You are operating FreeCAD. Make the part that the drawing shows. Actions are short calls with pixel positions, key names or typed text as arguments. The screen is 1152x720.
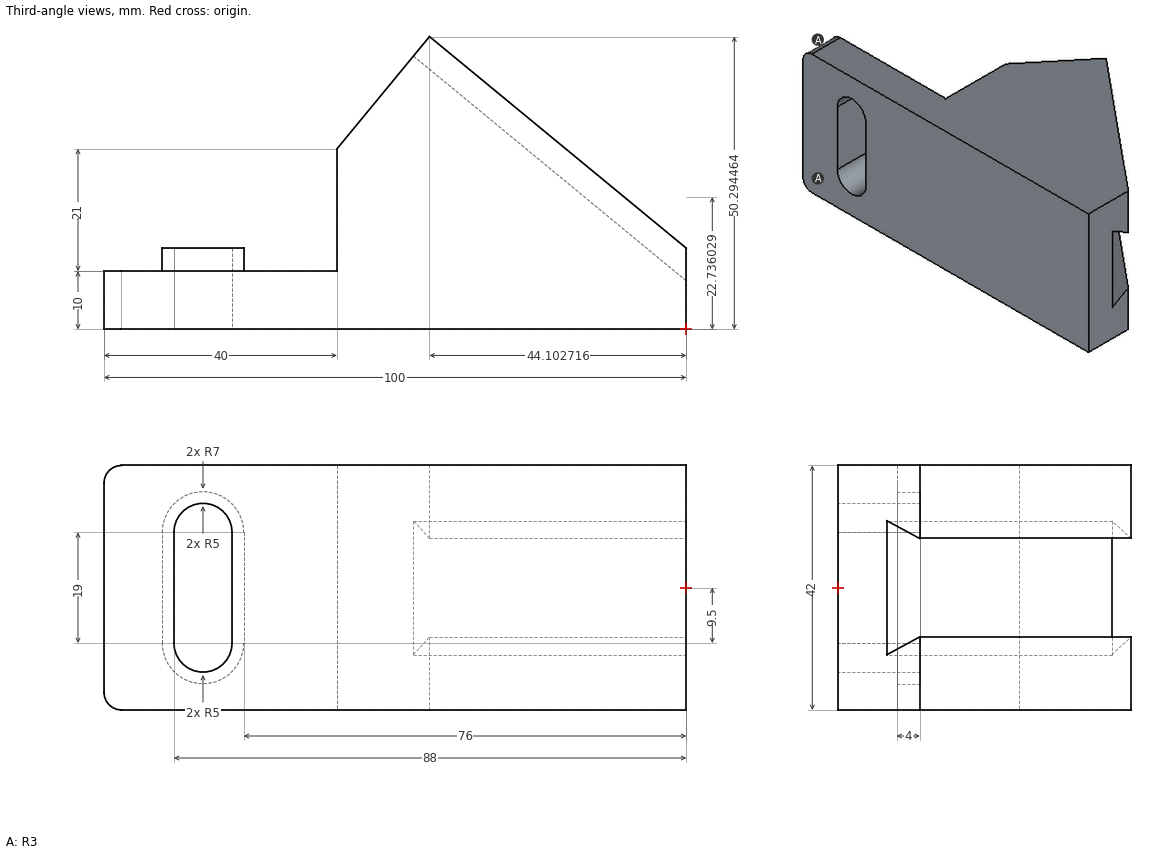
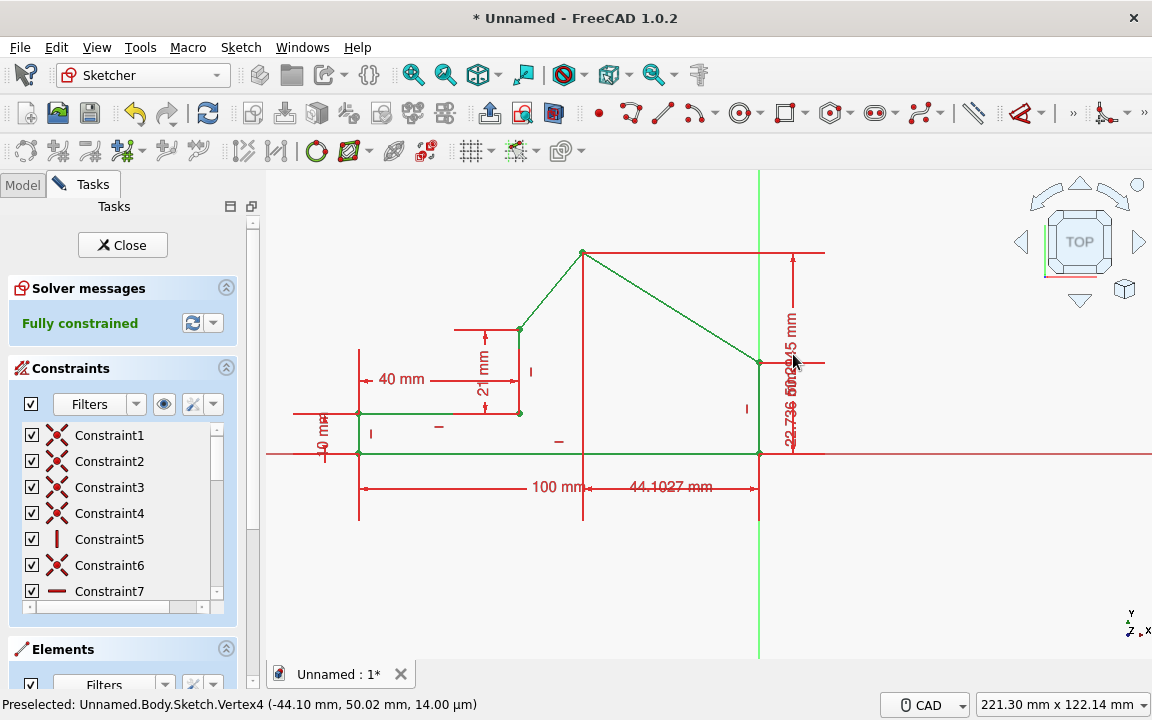
click(123, 245)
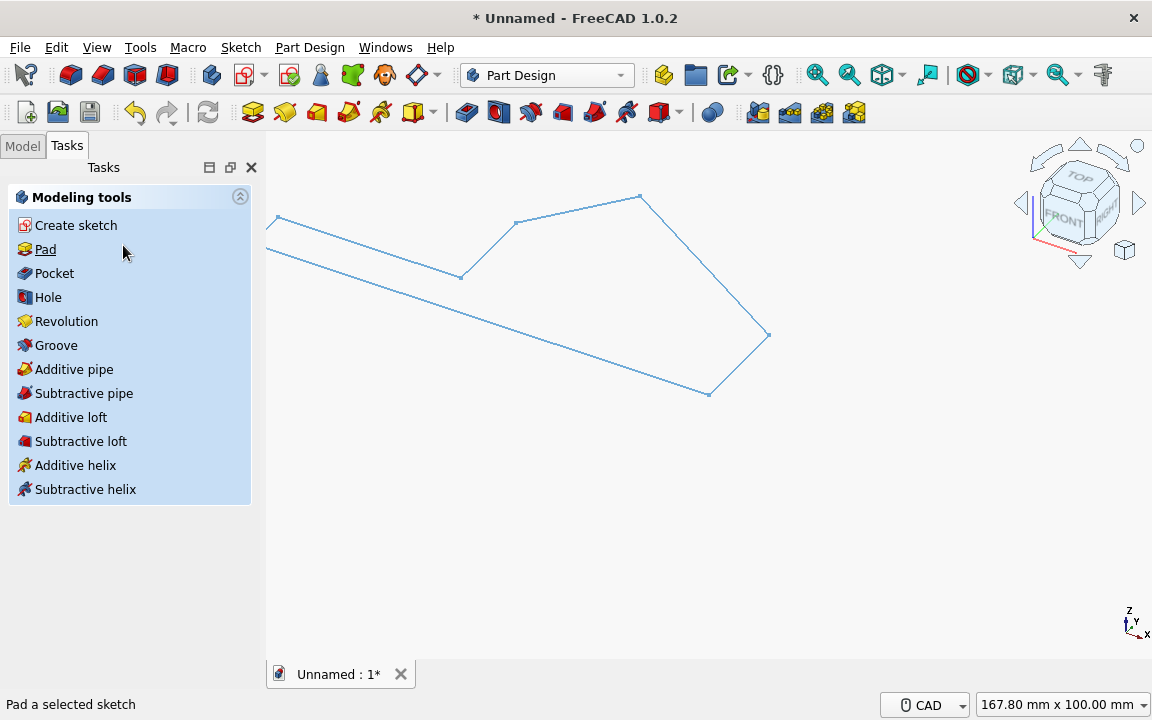
click(254, 112)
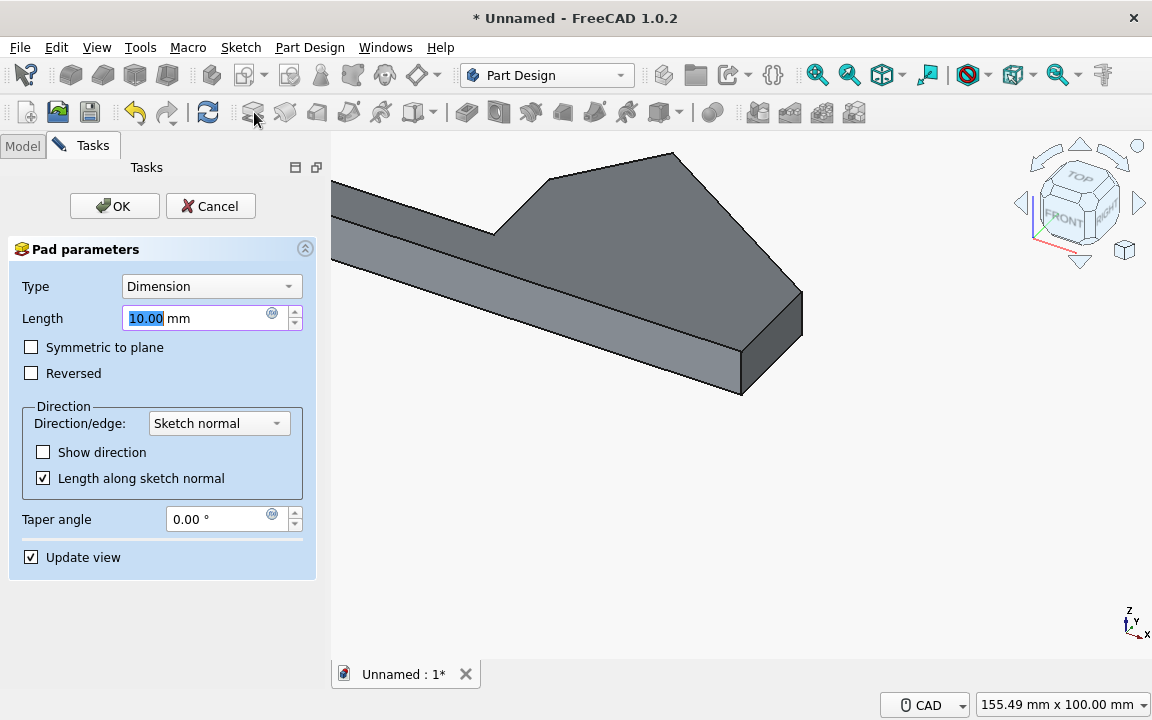
text(42)
key(Tab)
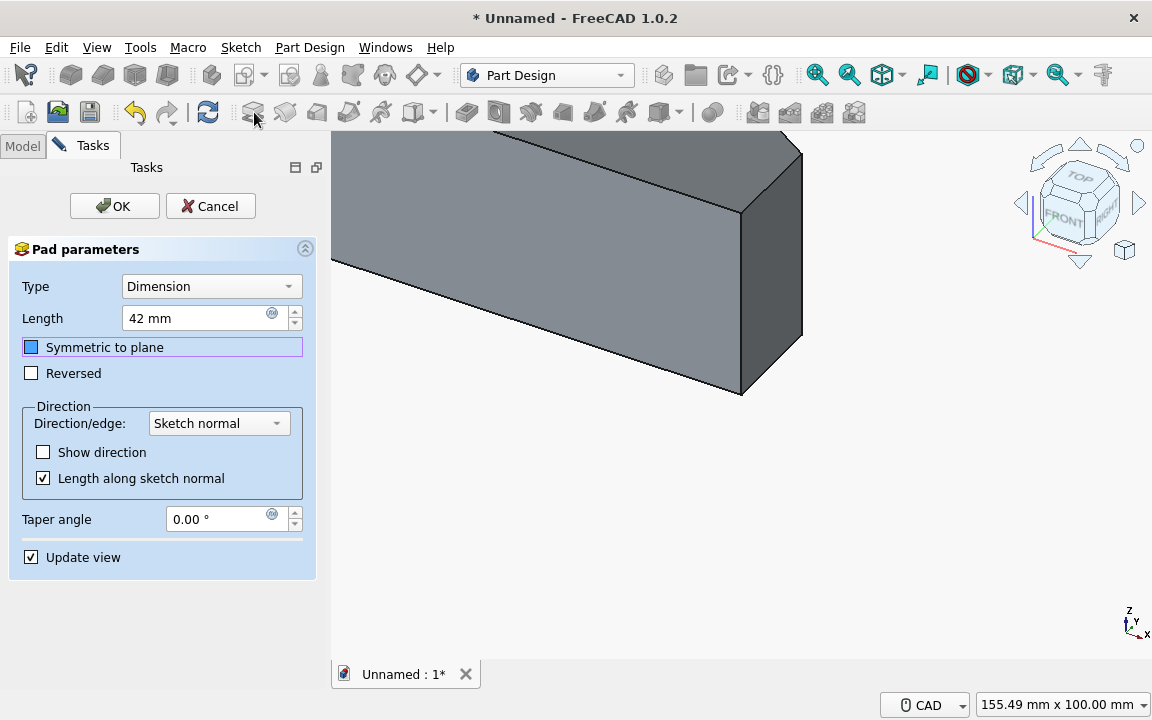
click(30, 347)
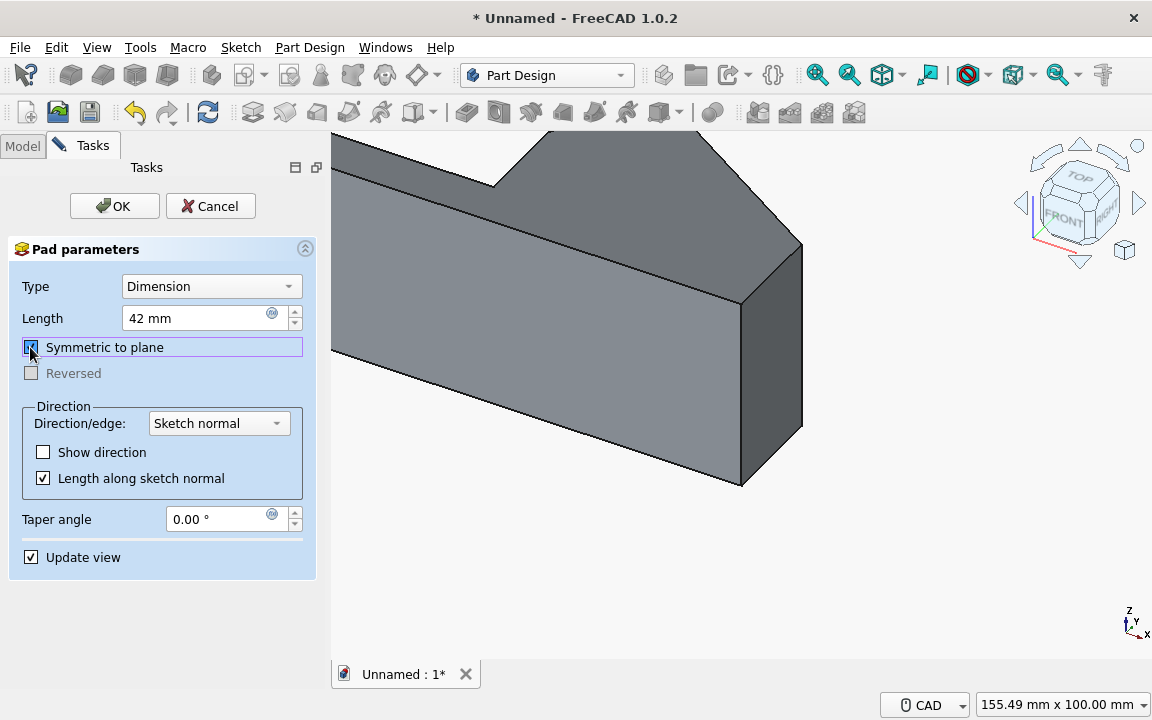
click(115, 206)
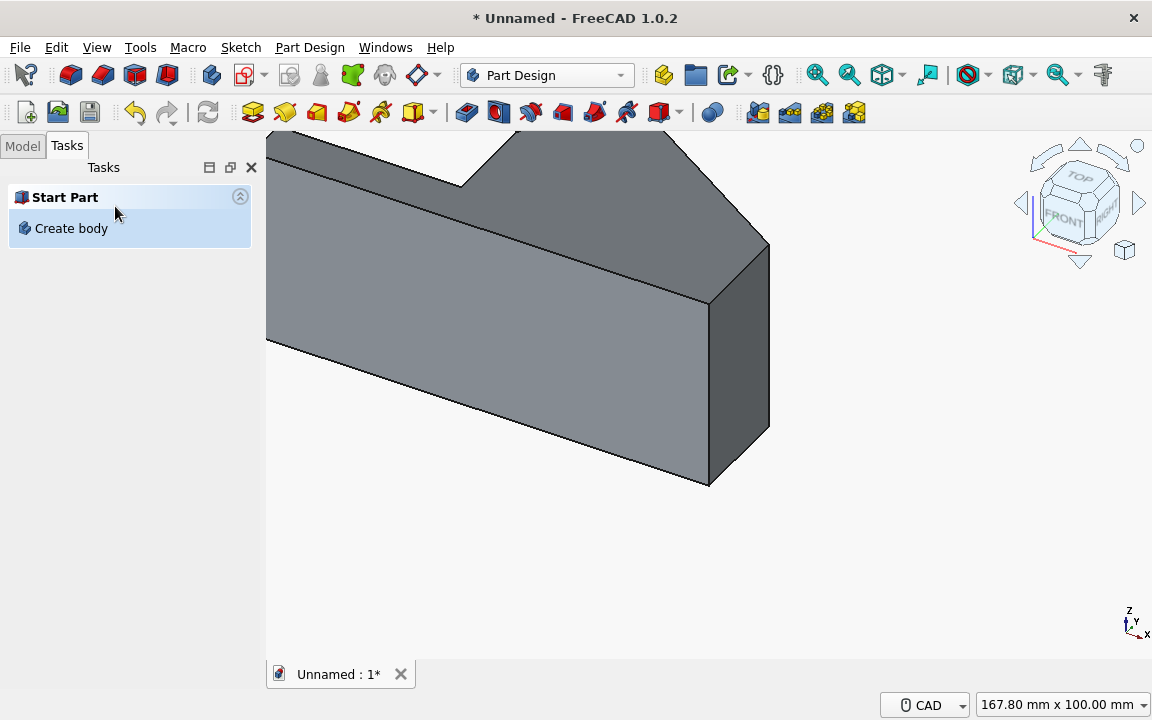
click(818, 76)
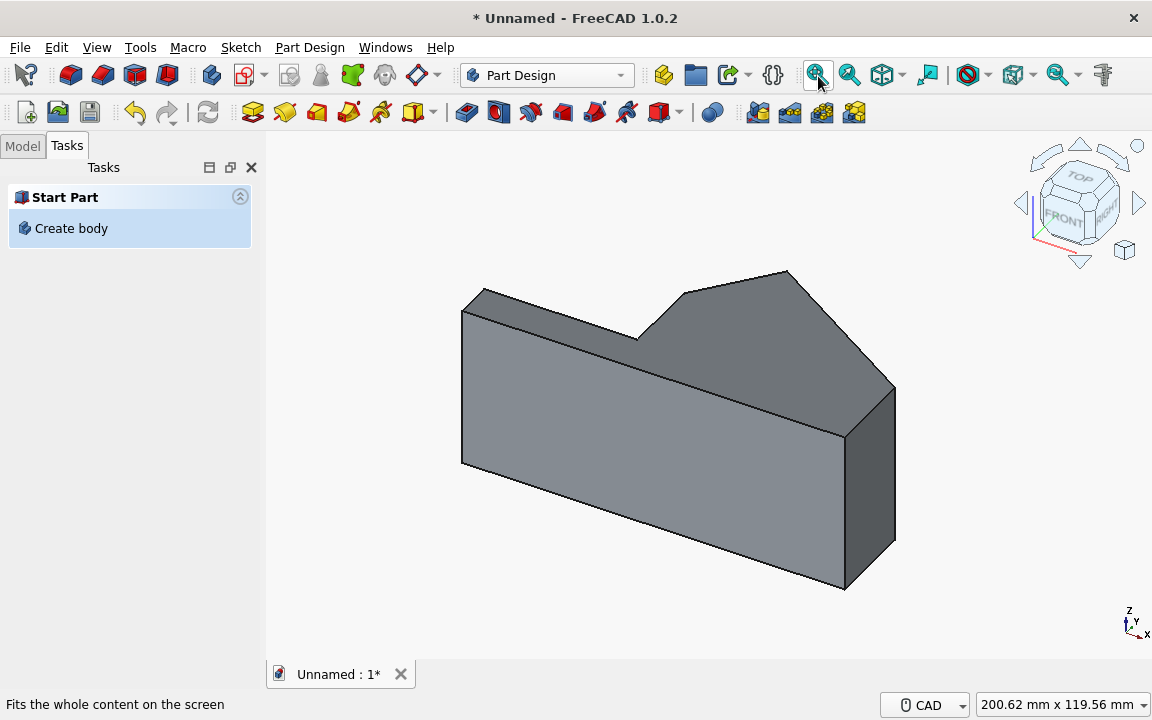
key(4)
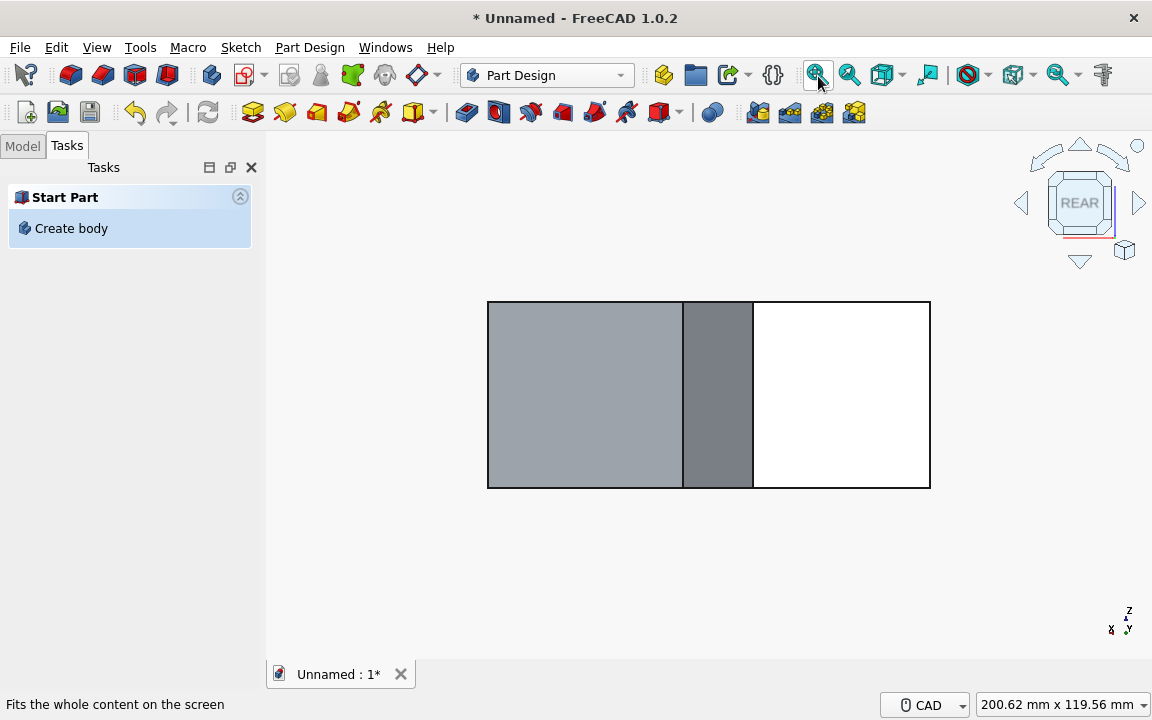
click(841, 394)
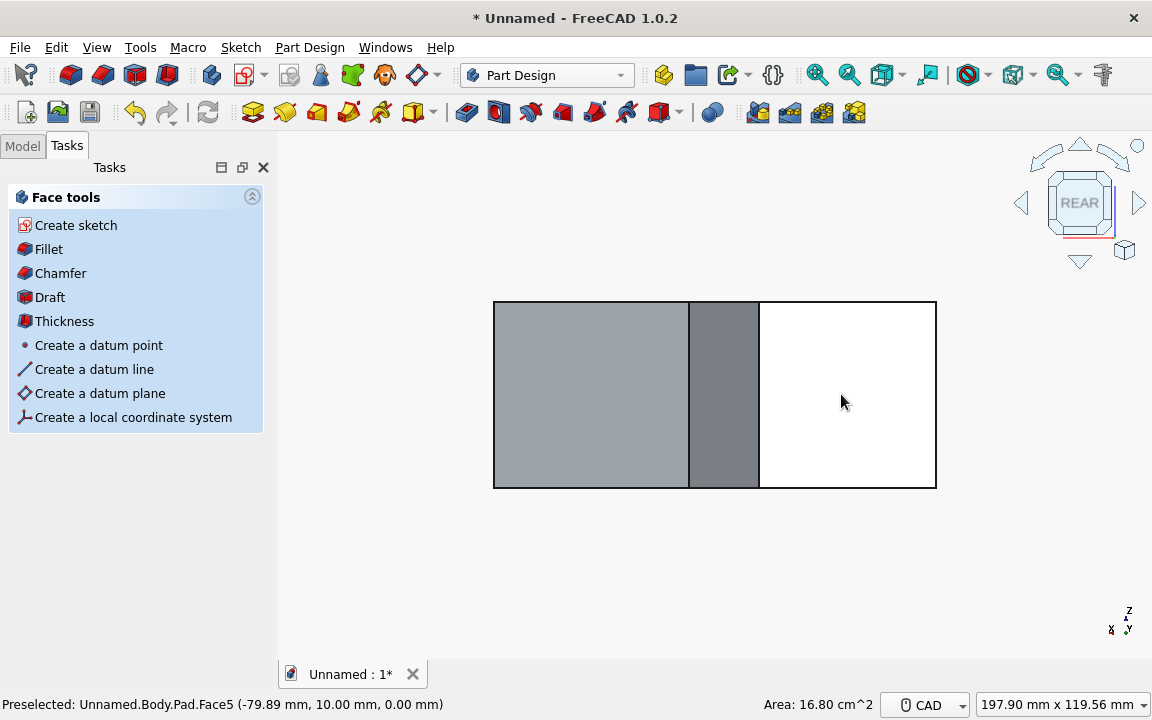
click(244, 76)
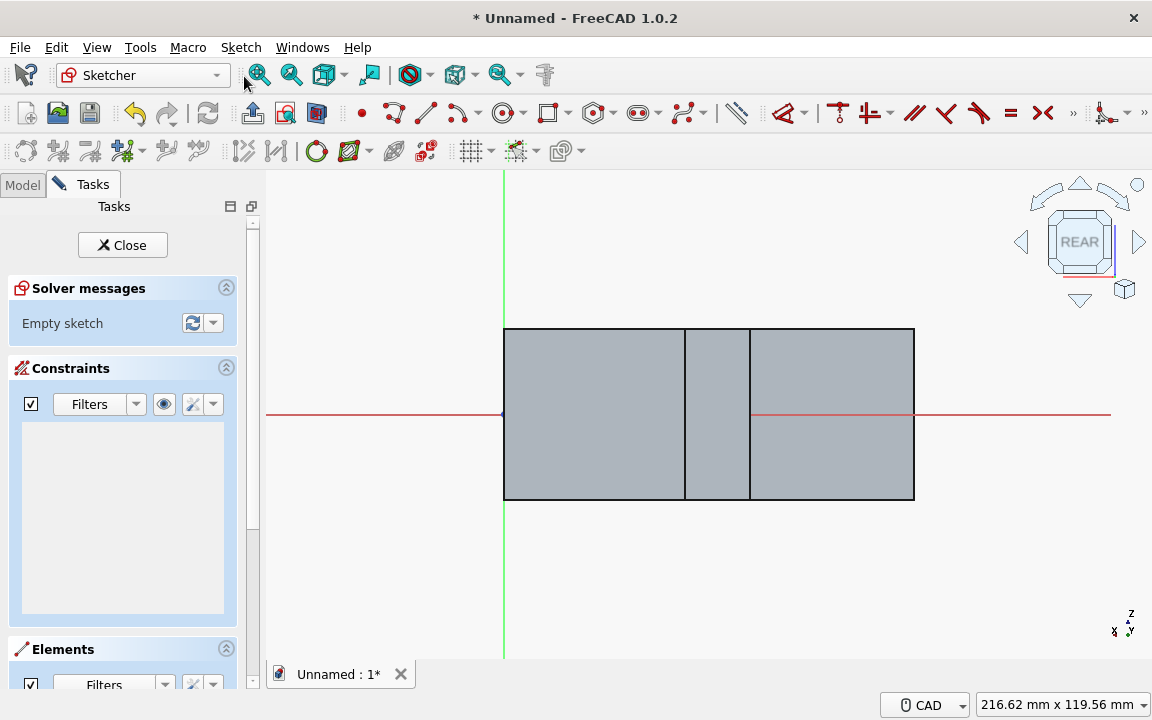
scroll(987, 414, up, 4)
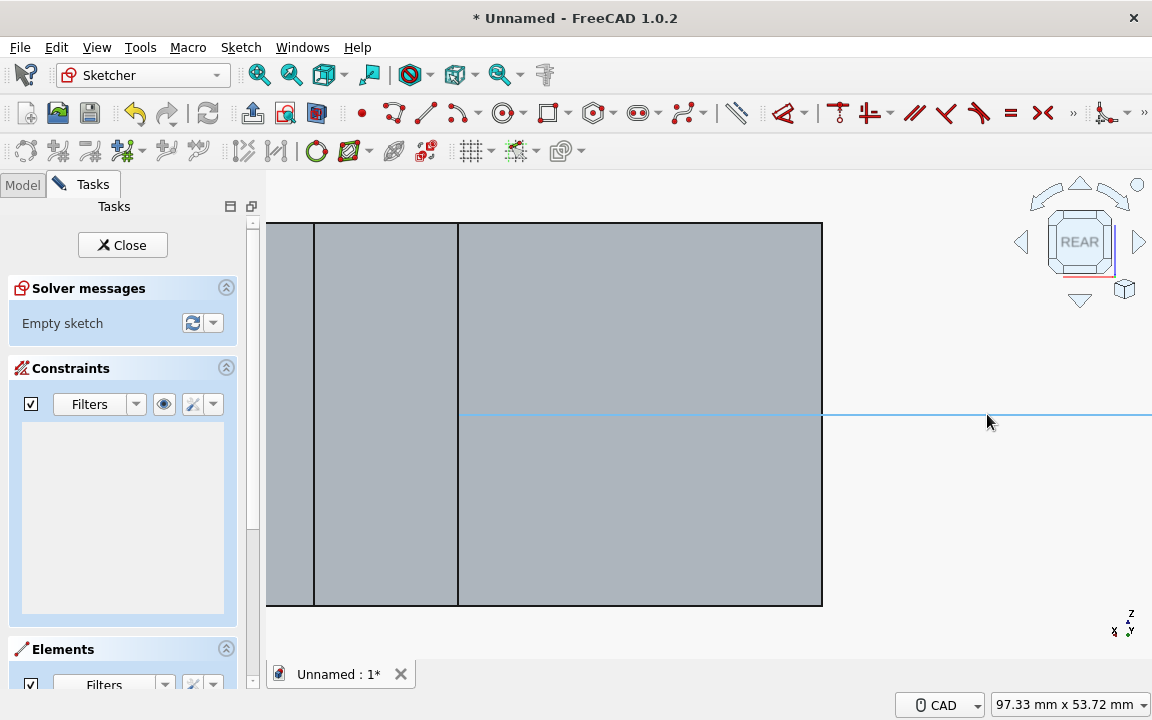
key(g)
key(s)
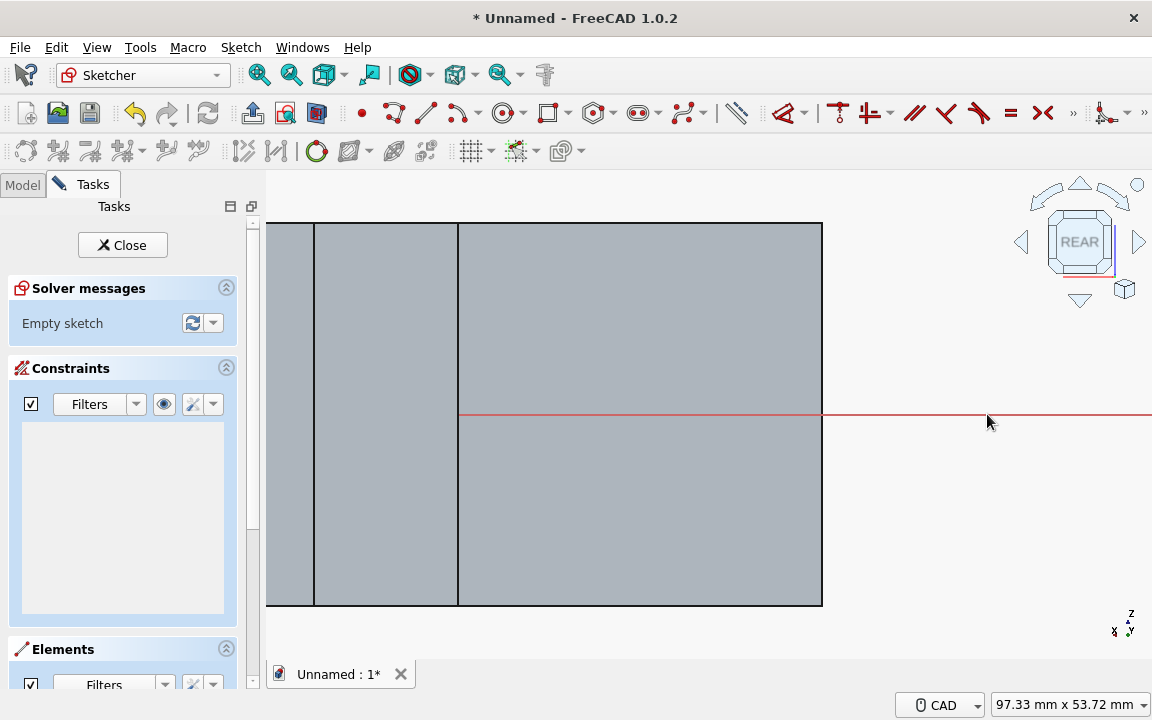
click(668, 501)